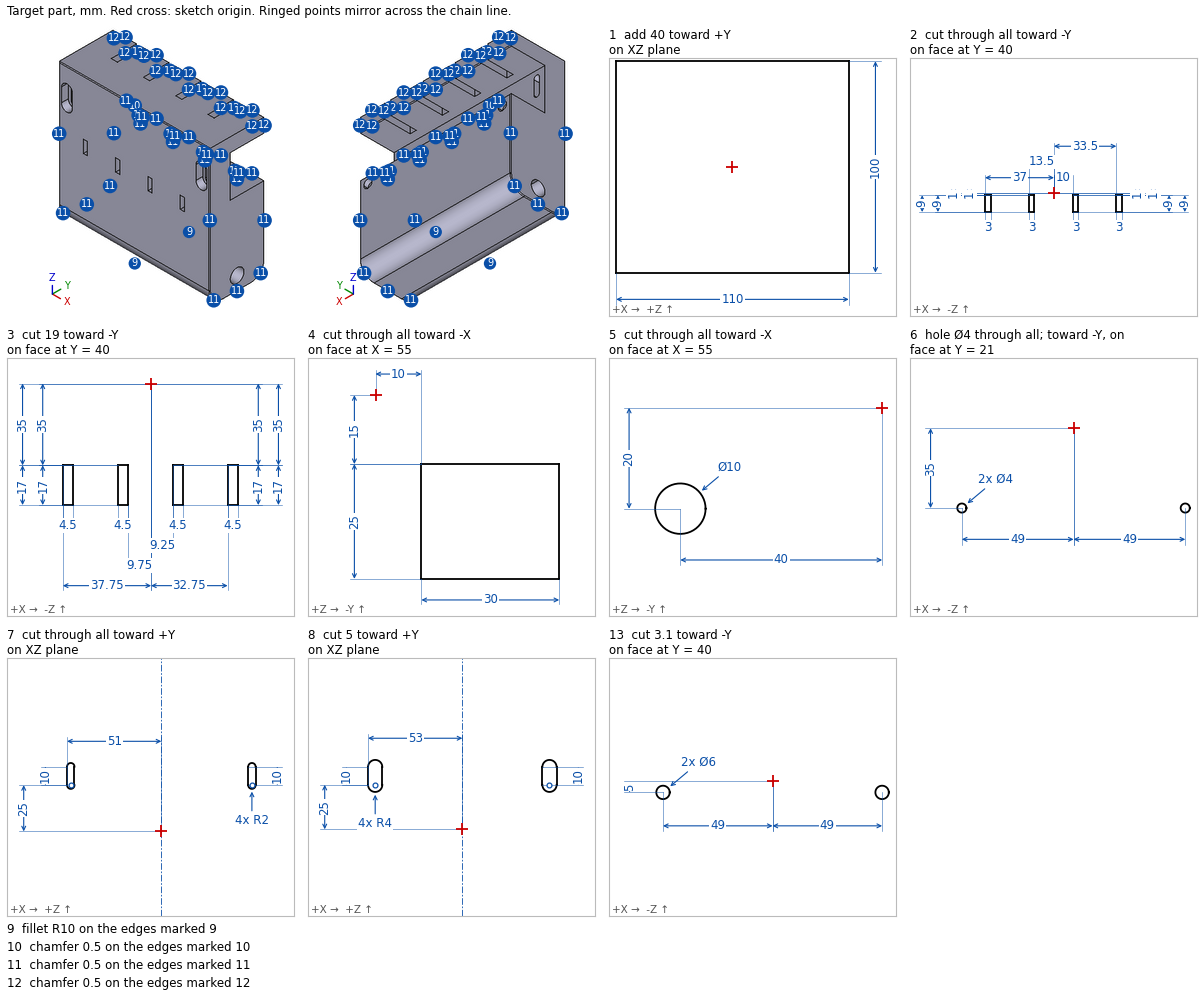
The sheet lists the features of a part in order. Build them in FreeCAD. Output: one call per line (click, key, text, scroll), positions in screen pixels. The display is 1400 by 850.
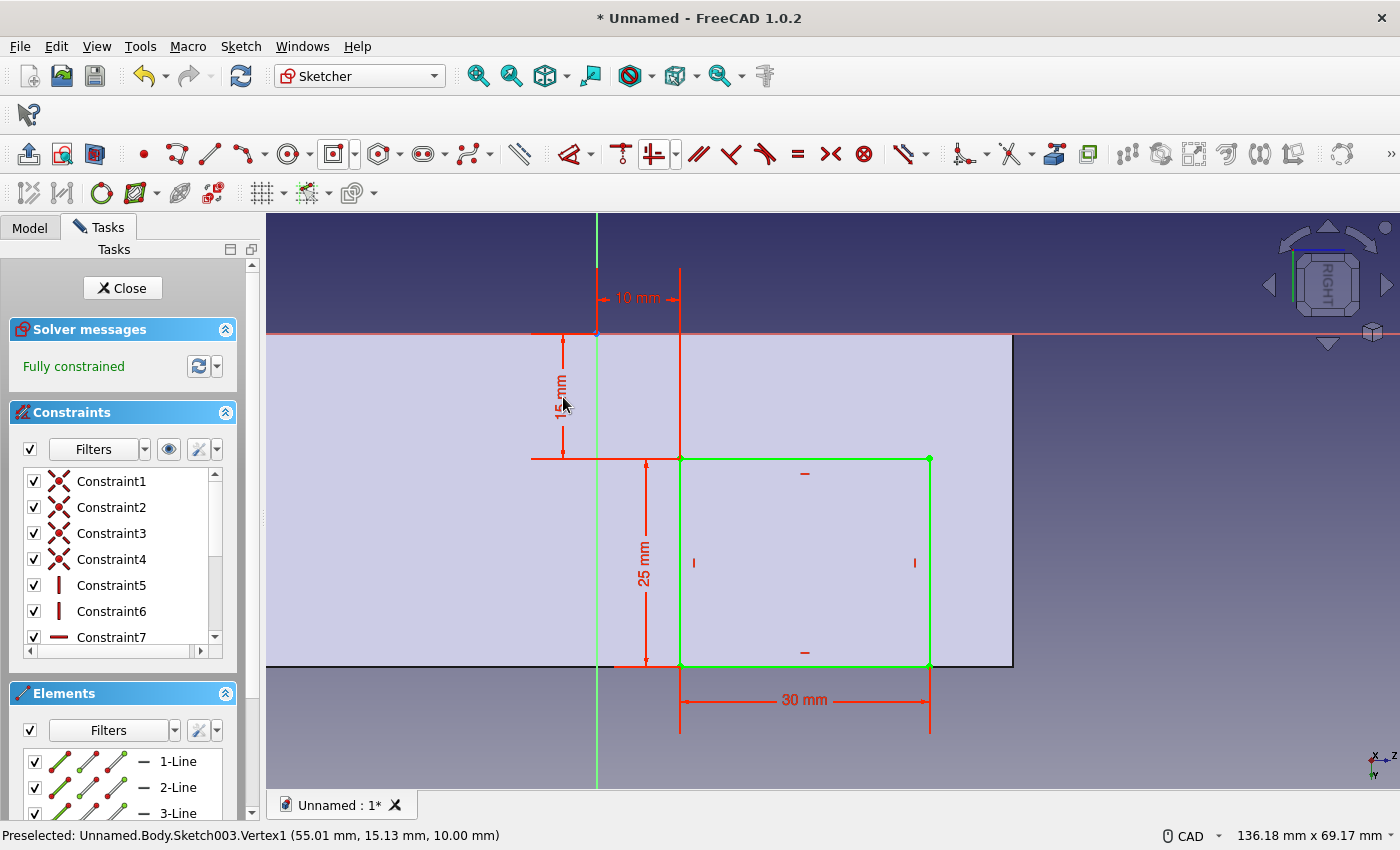
click(123, 288)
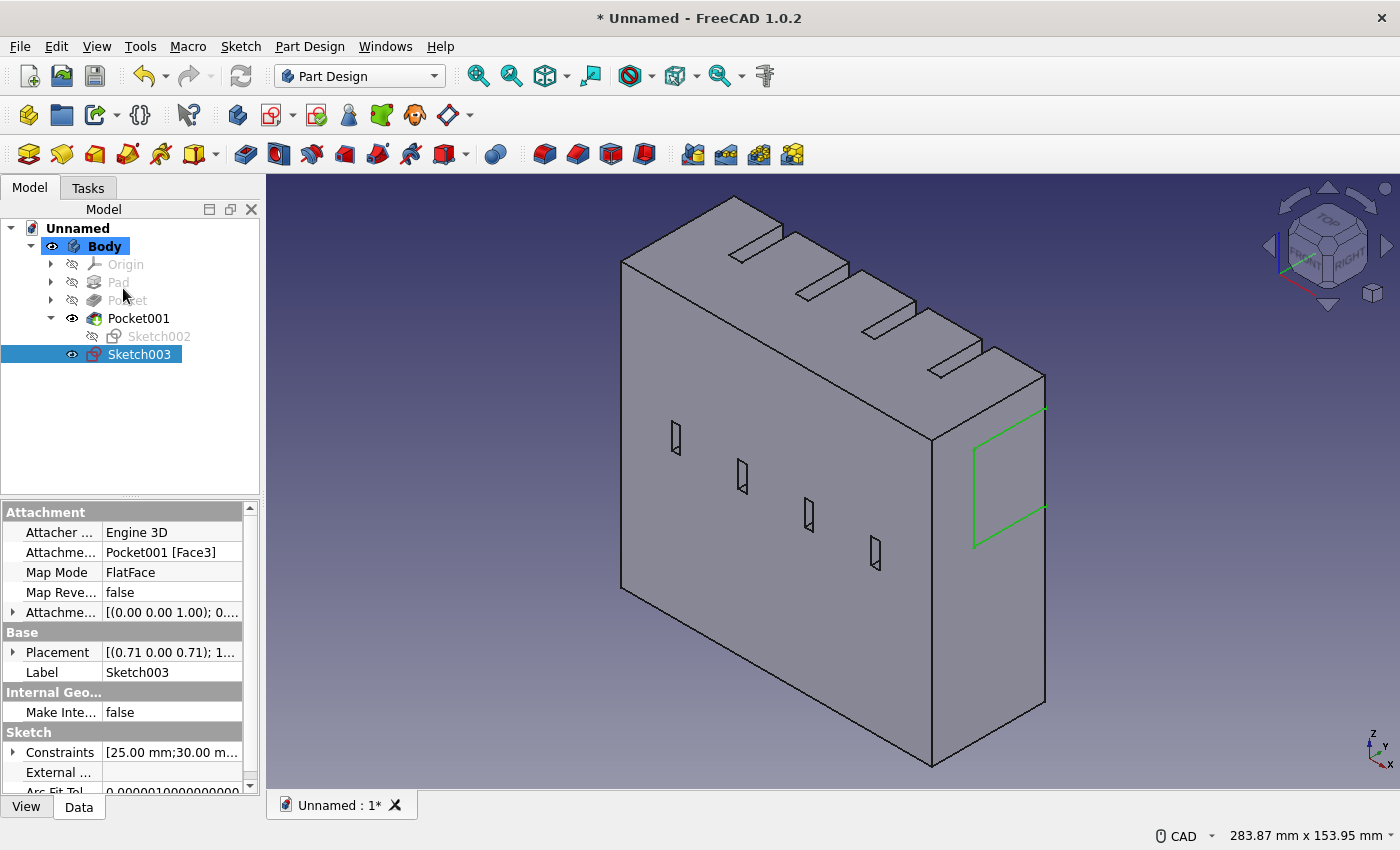
click(246, 154)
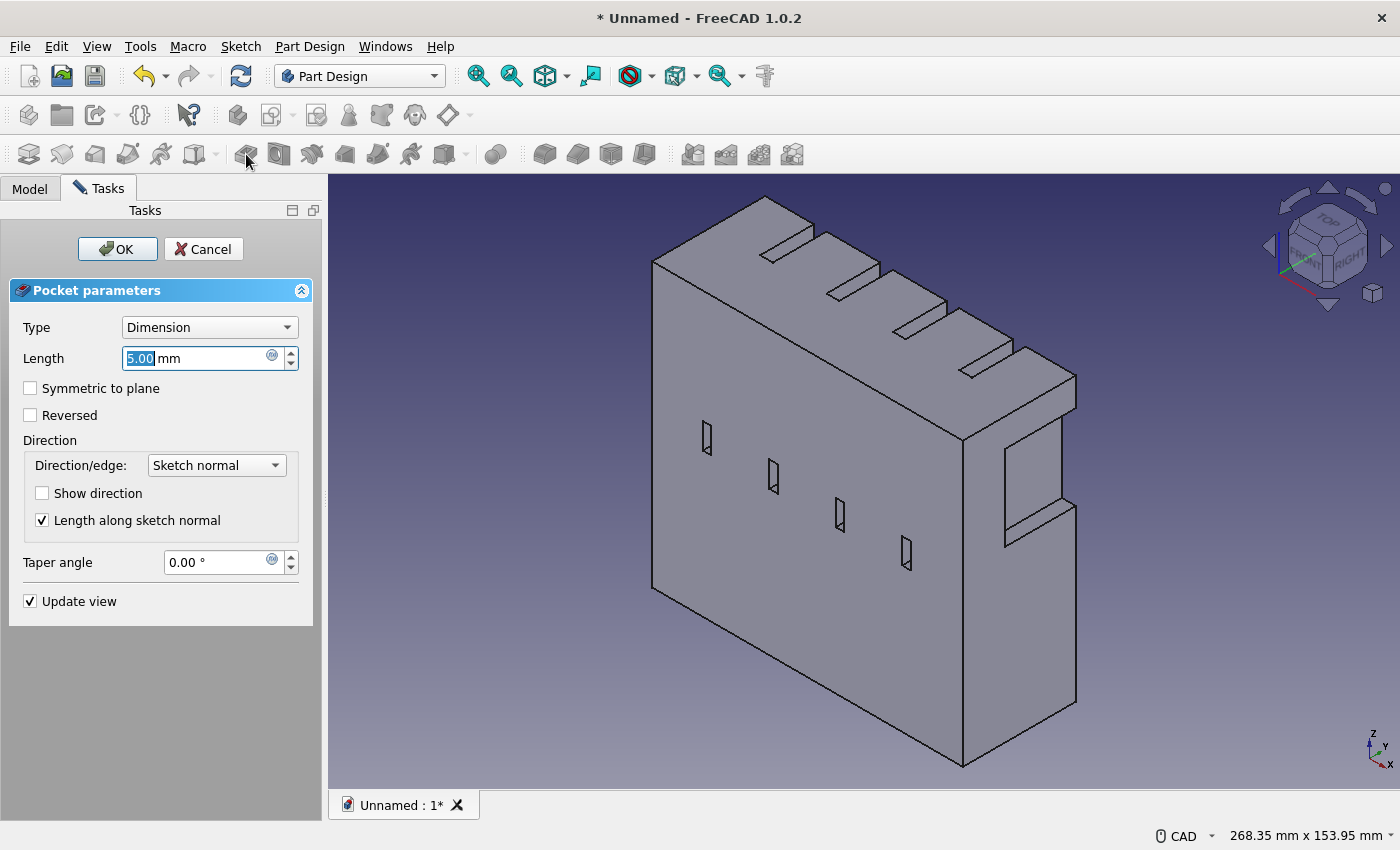
click(210, 328)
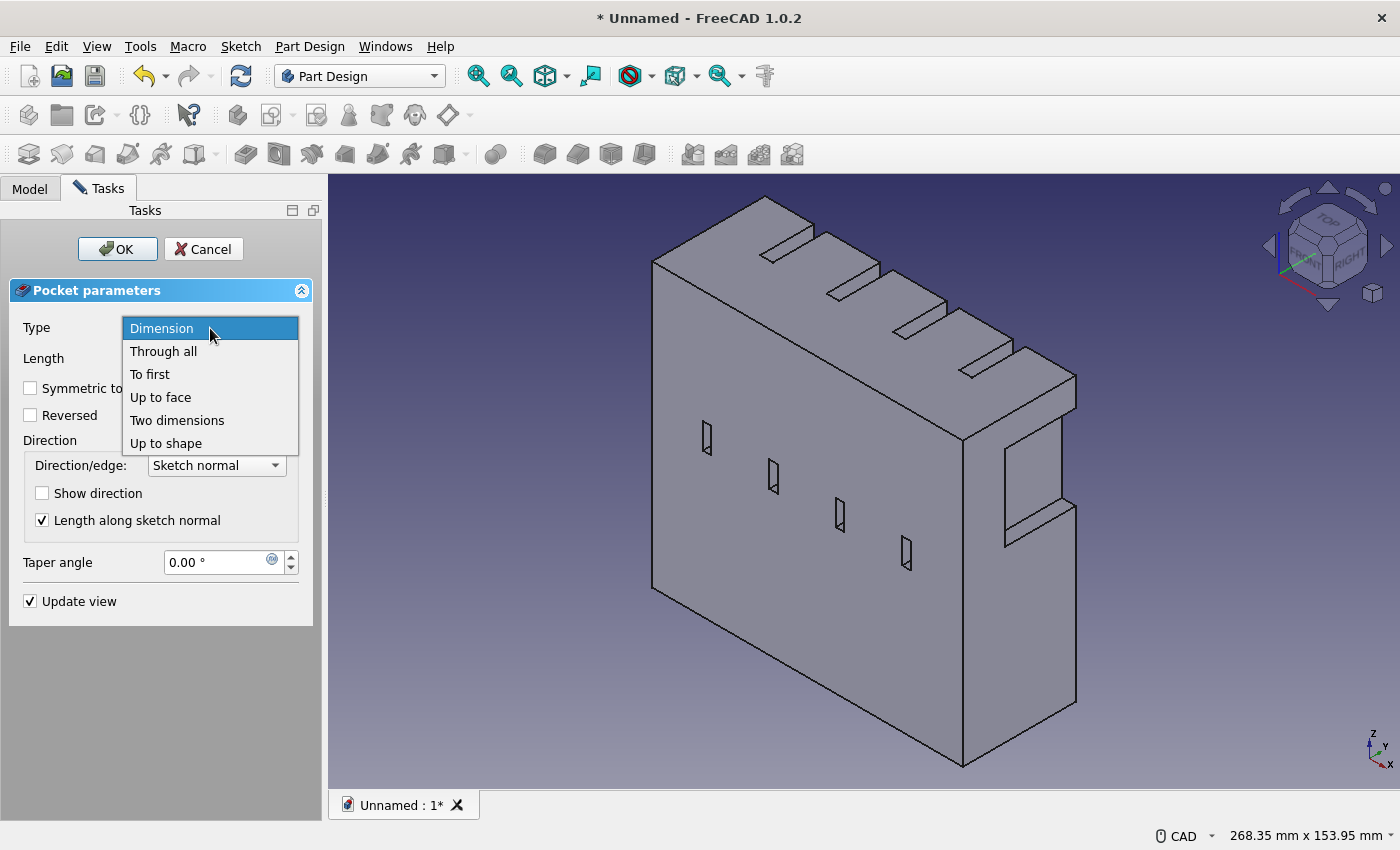
click(208, 352)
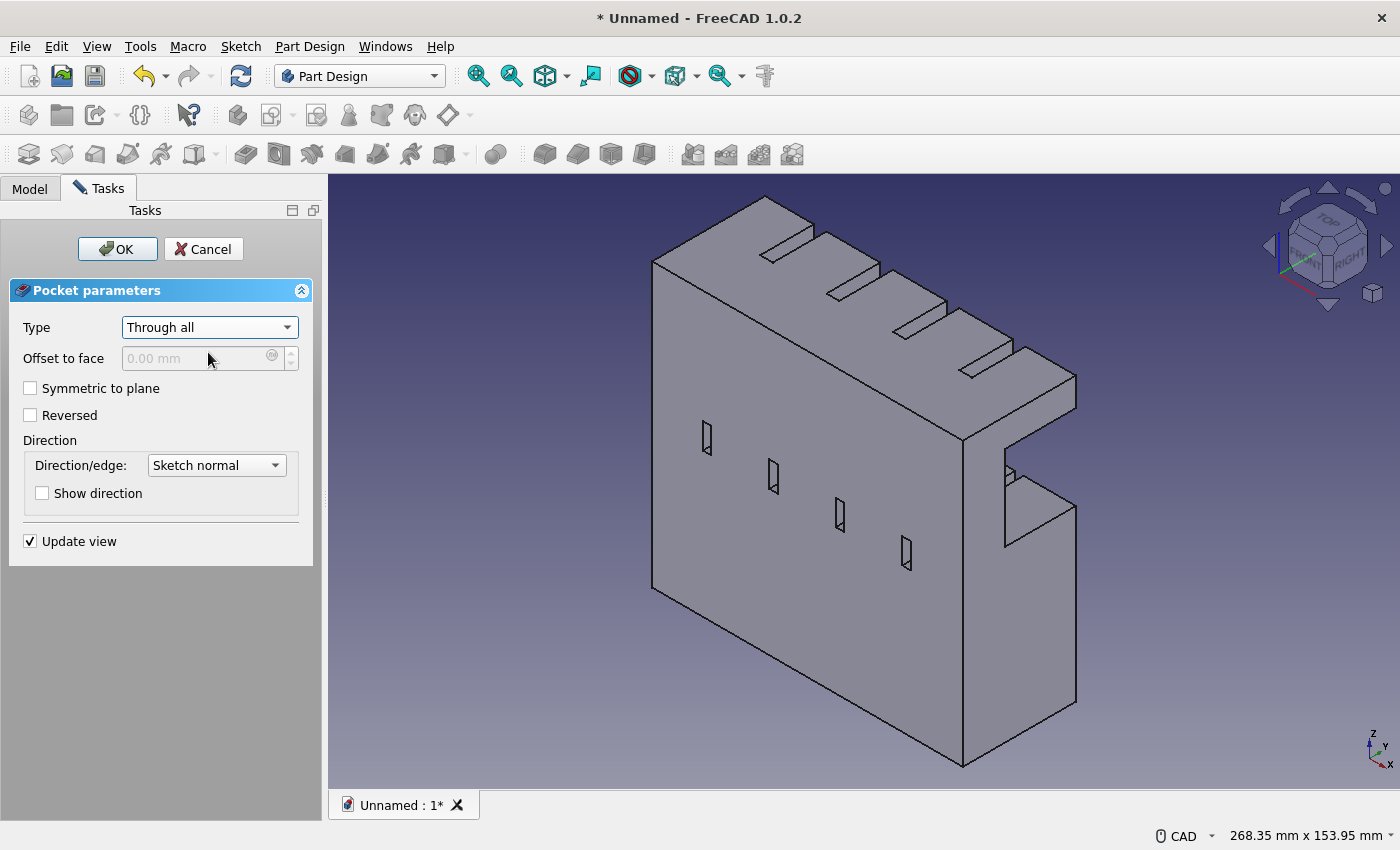
click(118, 249)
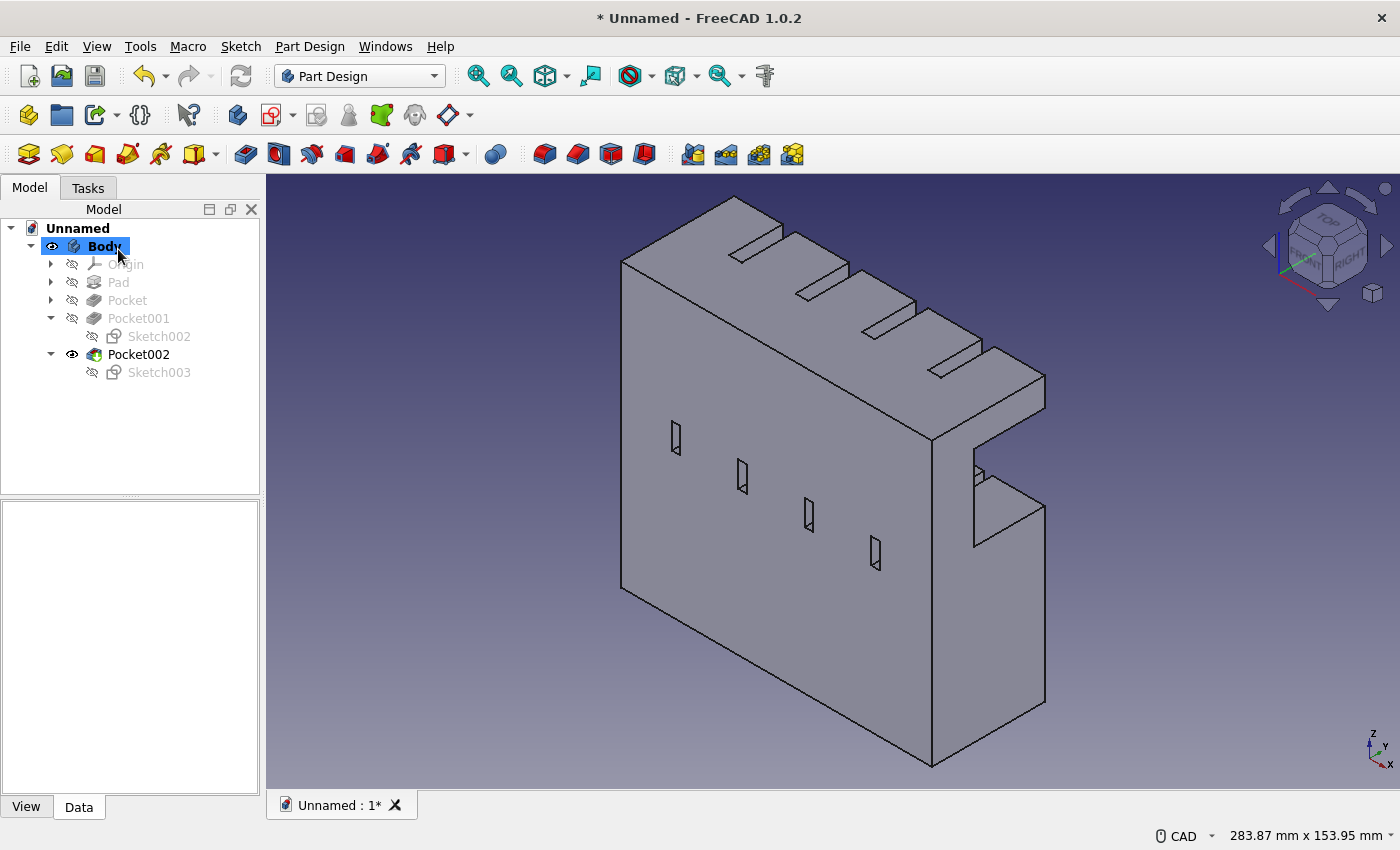
click(988, 617)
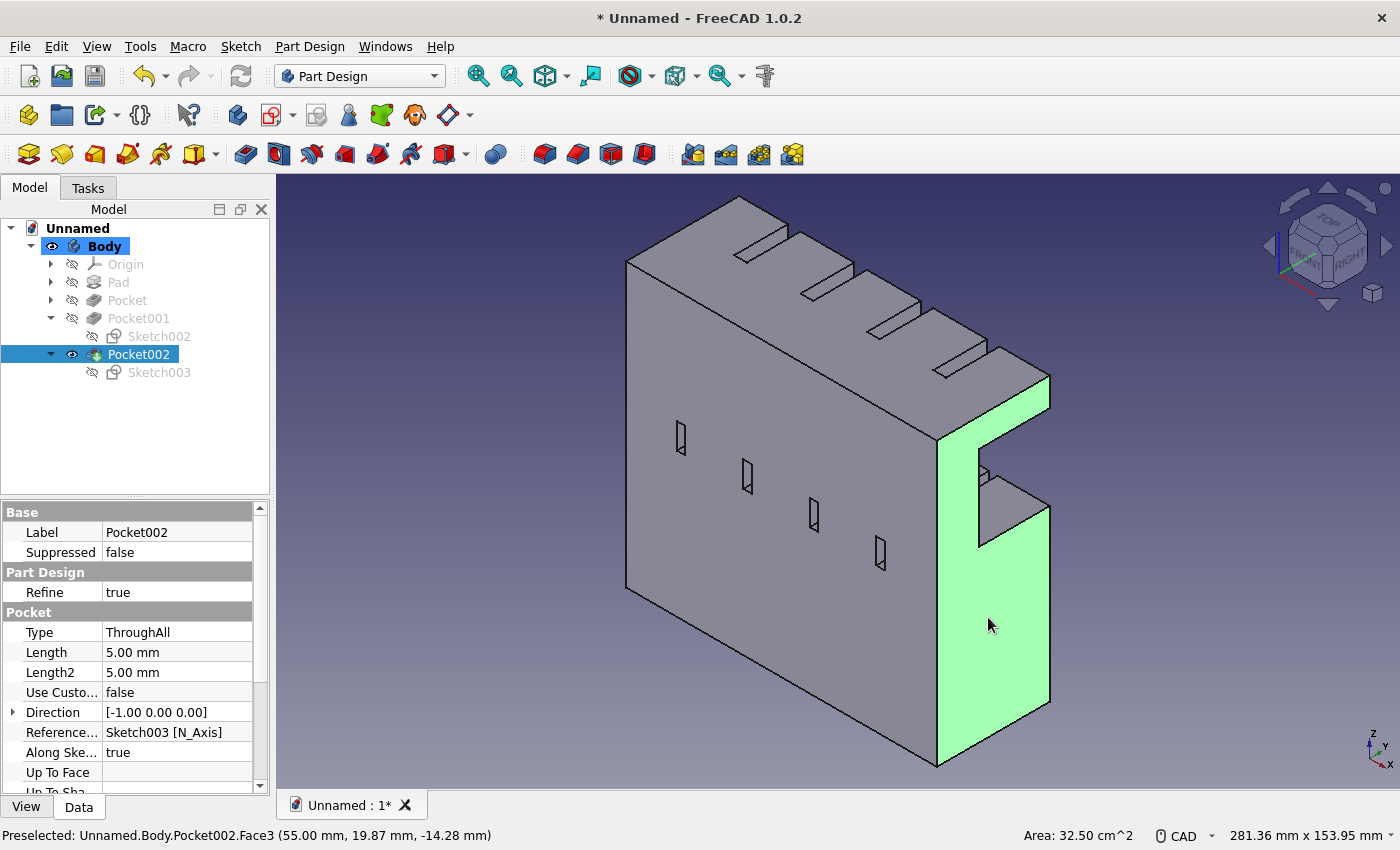
click(270, 116)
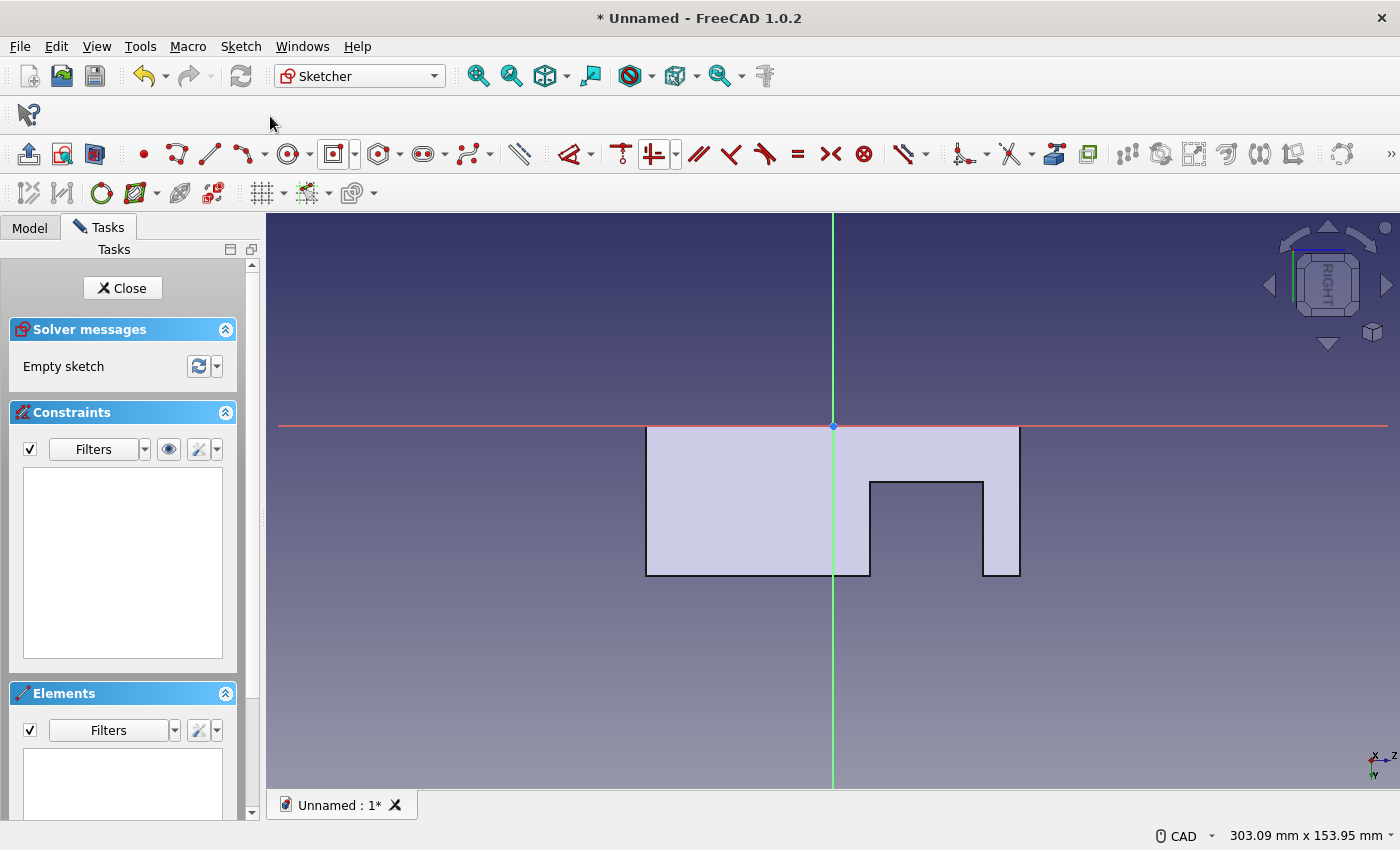
scroll(673, 501, up, 11)